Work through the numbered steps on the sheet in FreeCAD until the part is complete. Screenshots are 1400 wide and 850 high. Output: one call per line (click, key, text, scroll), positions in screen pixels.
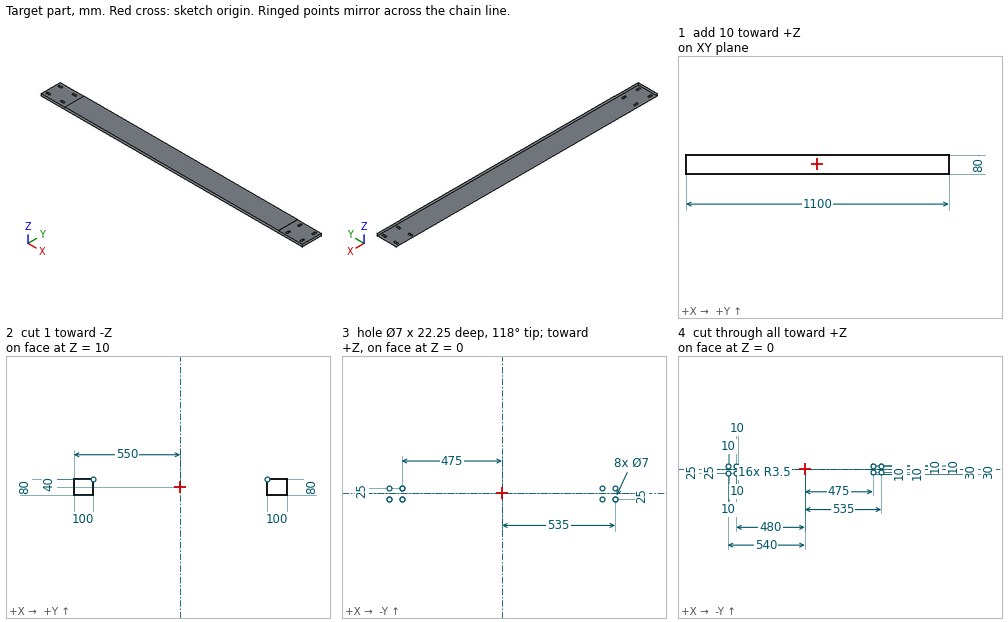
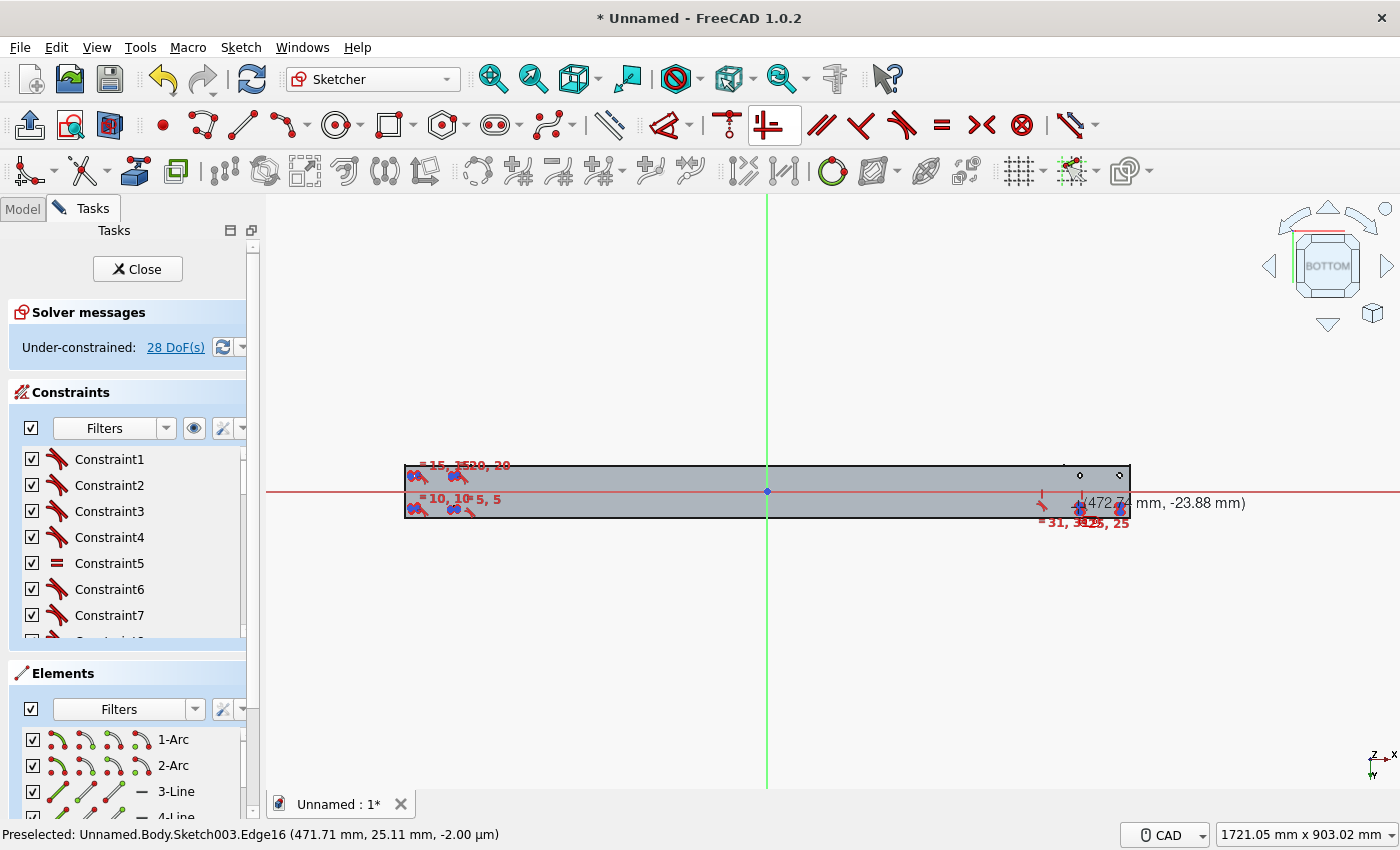
scroll(1120, 479, up, 12)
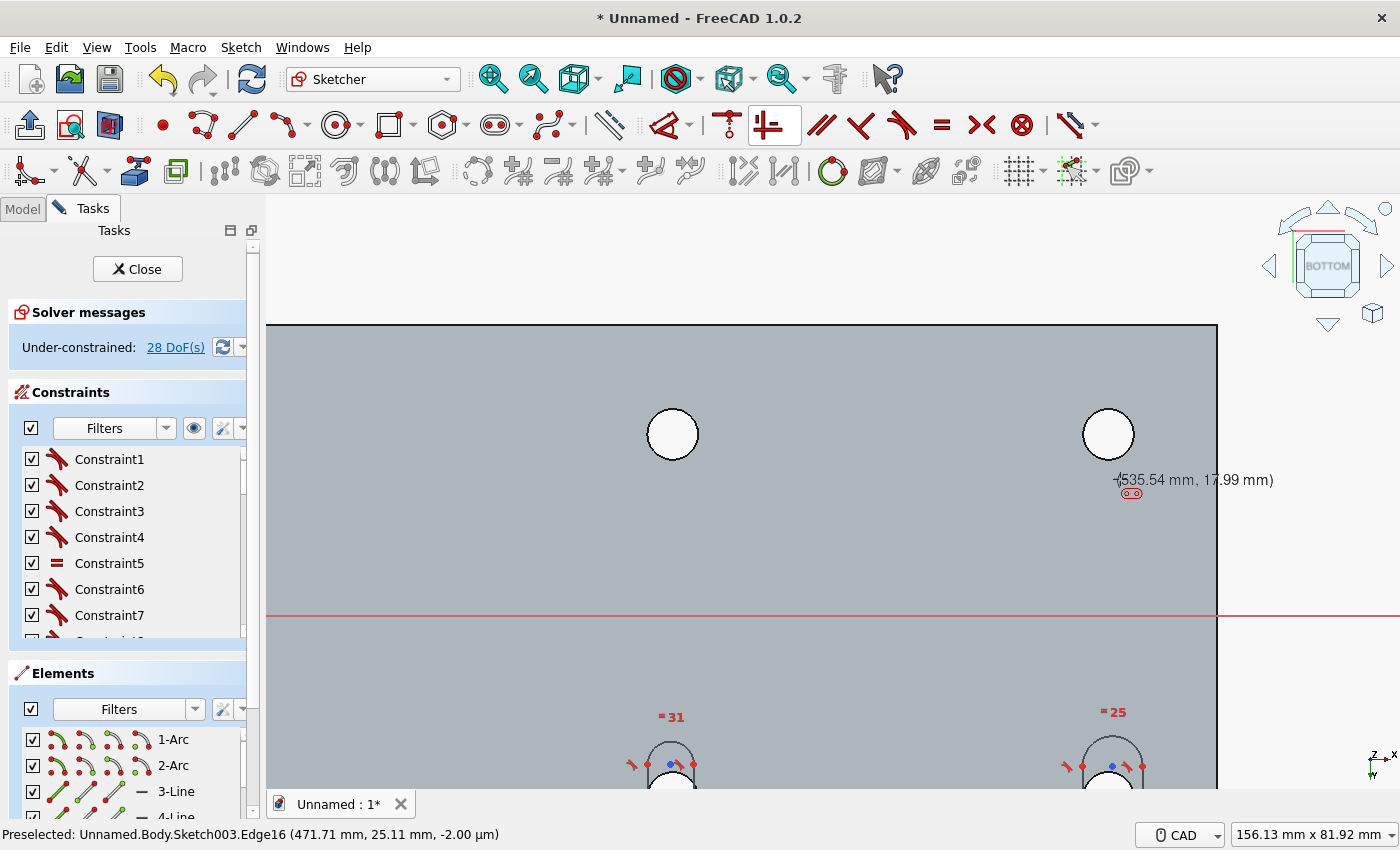
scroll(1120, 479, down, 12)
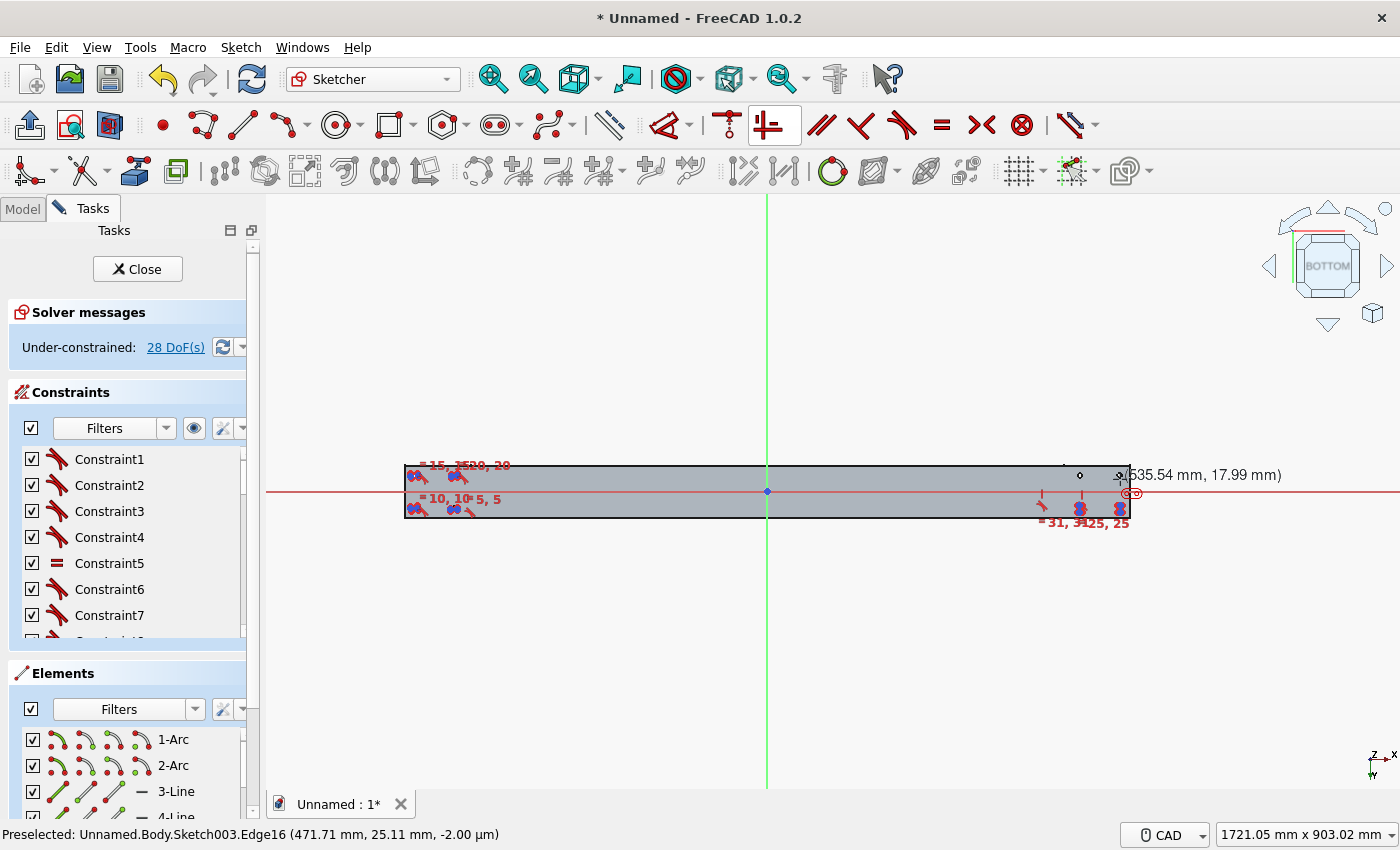
click(1120, 479)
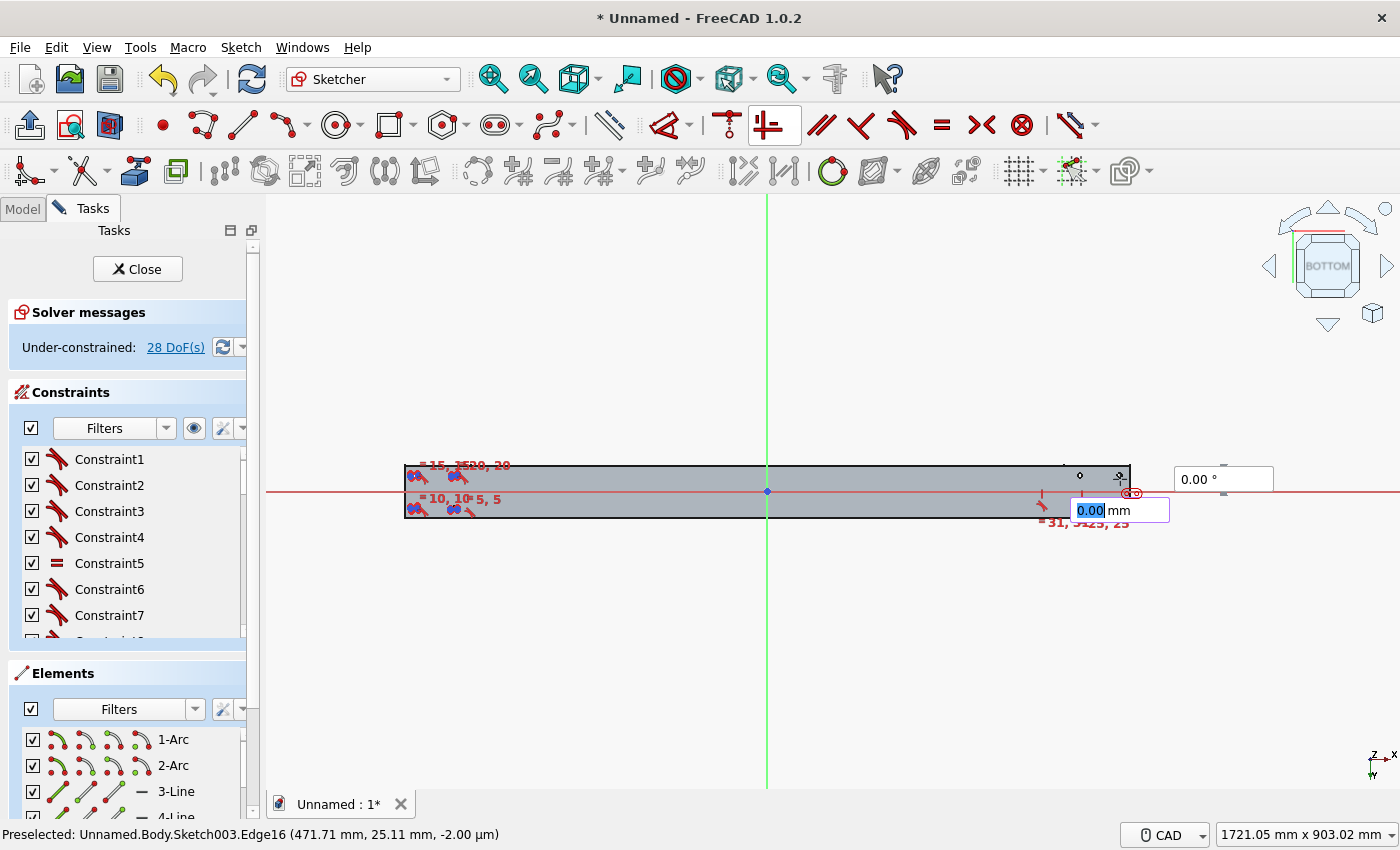
scroll(1120, 472, up, 5)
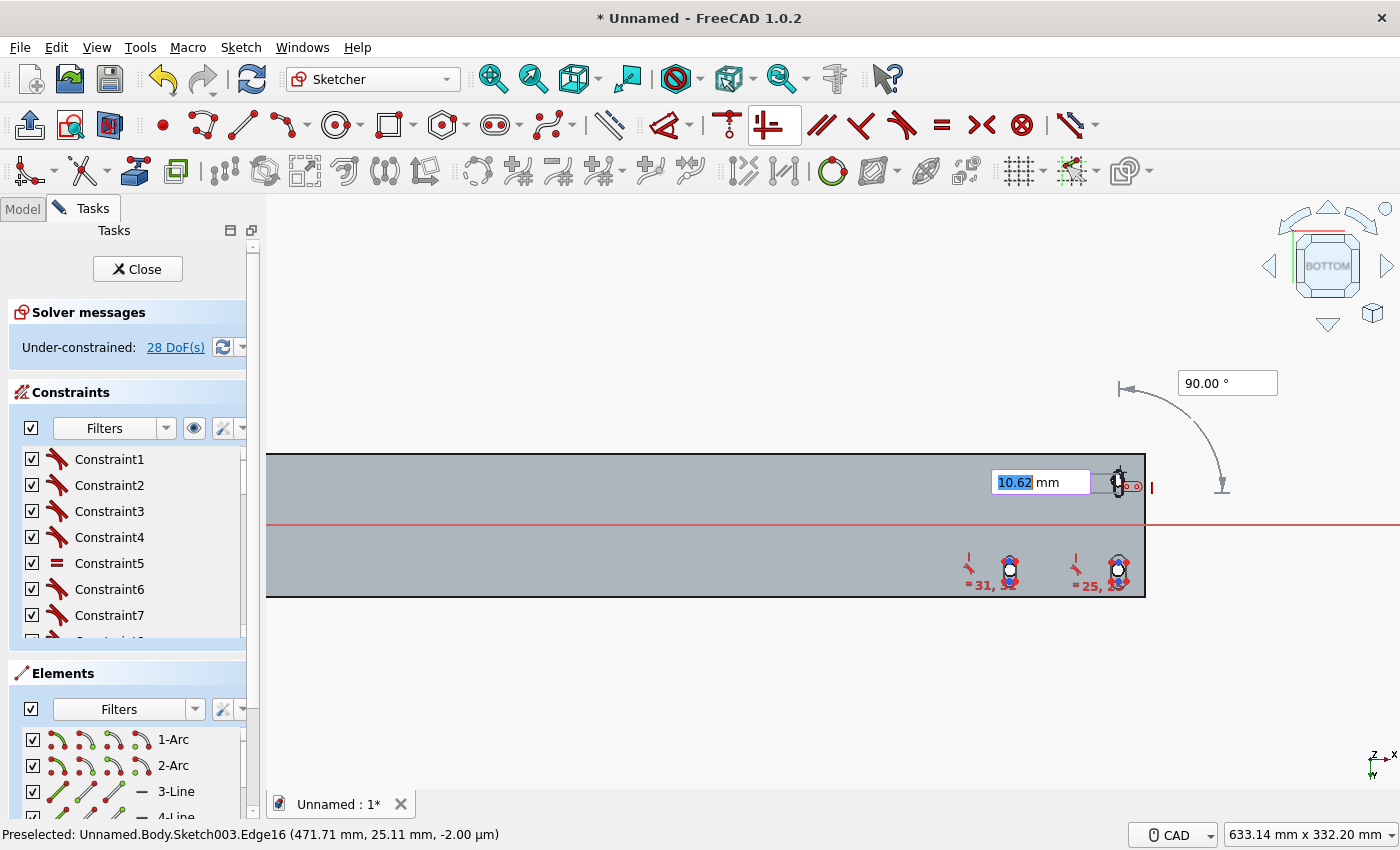
click(1119, 471)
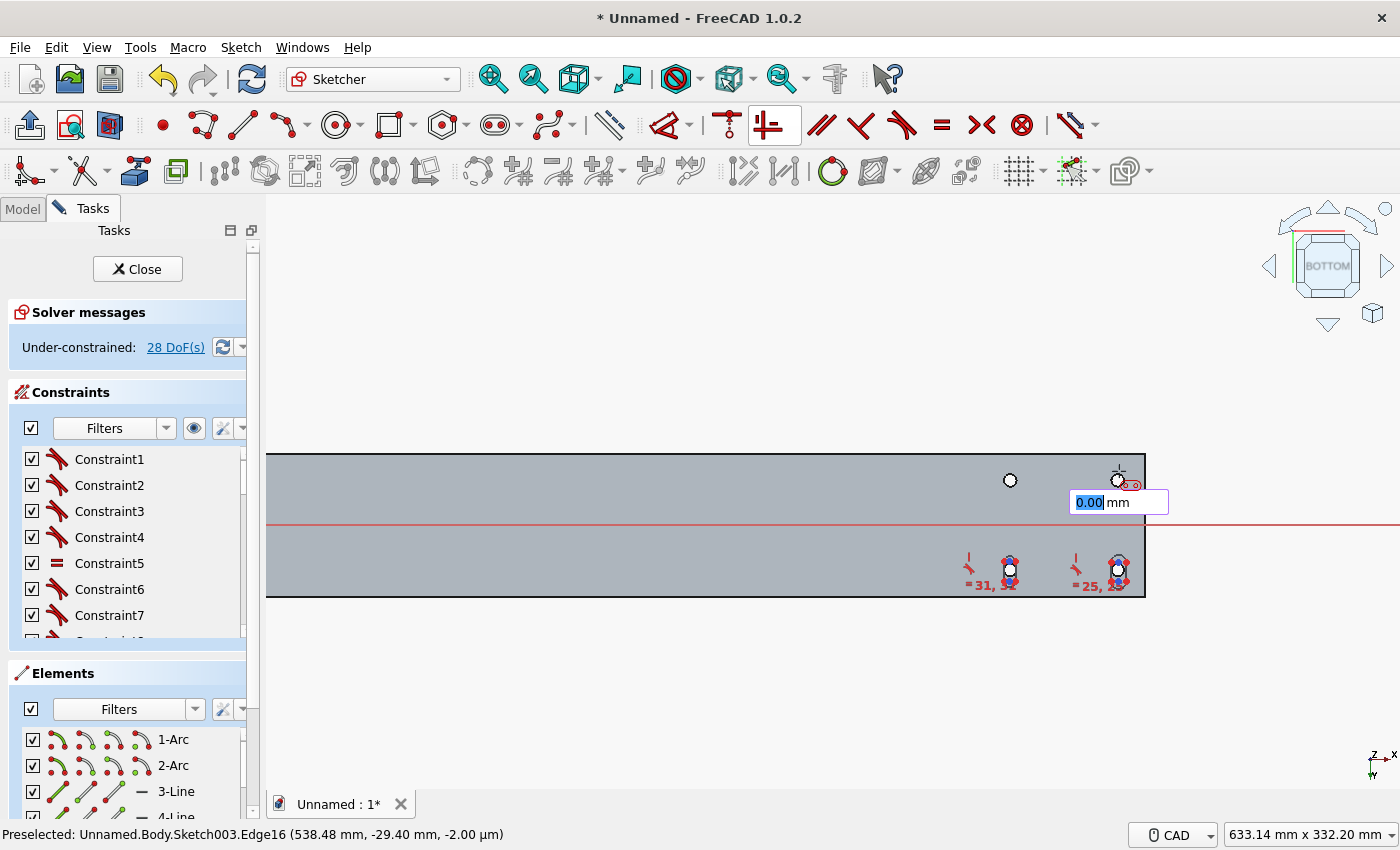
scroll(1124, 480, up, 5)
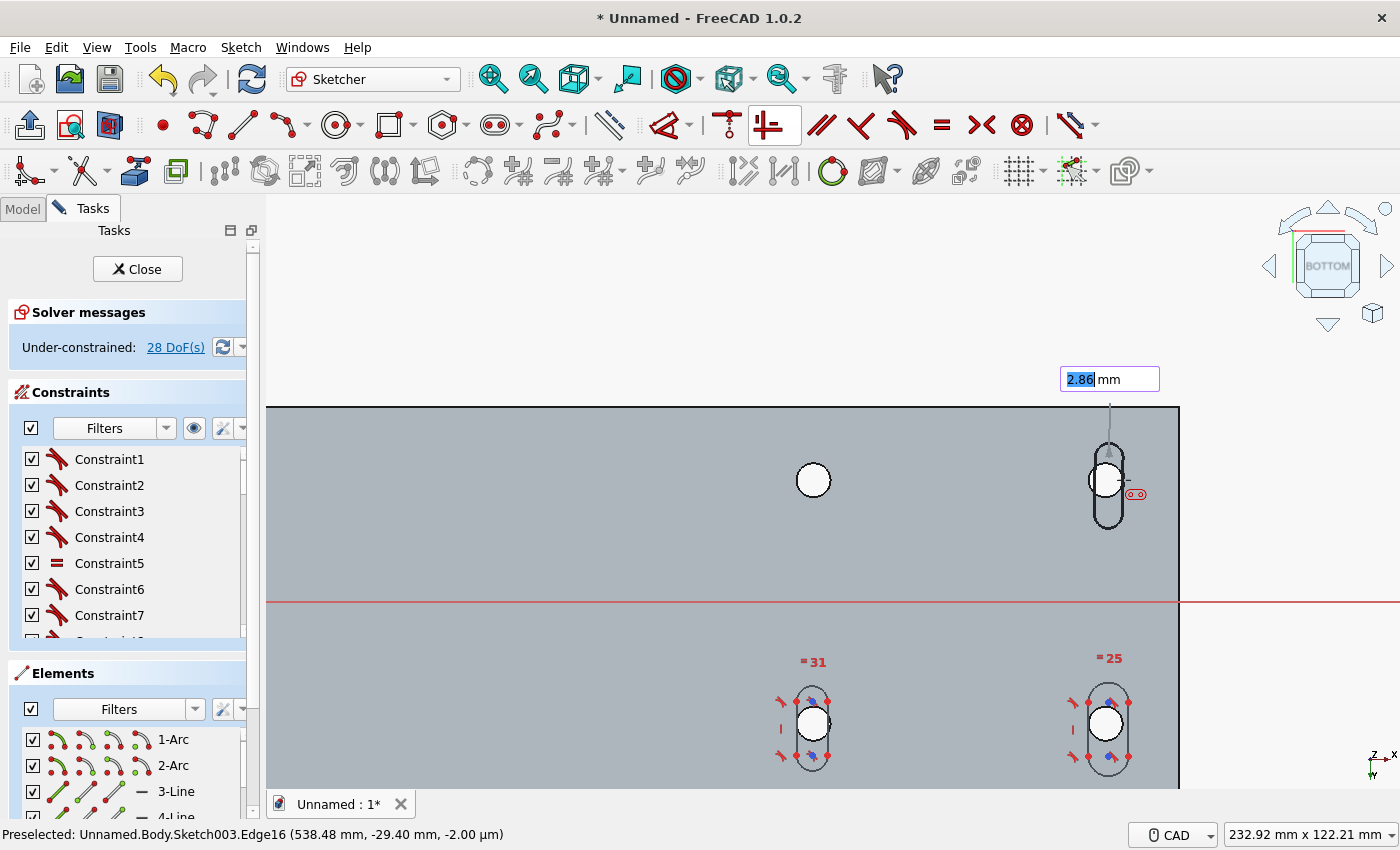
click(1123, 480)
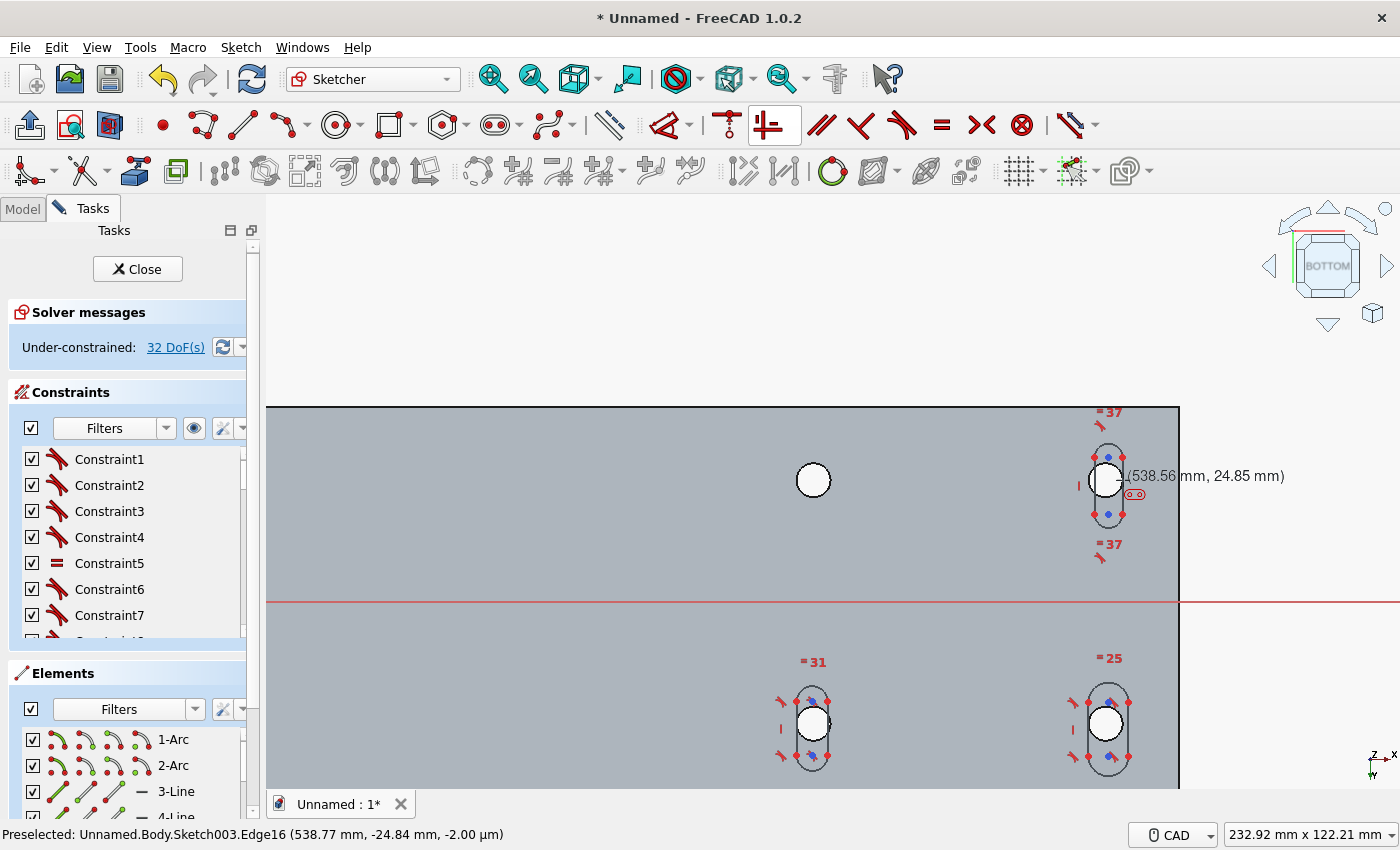
scroll(814, 505, up, 2)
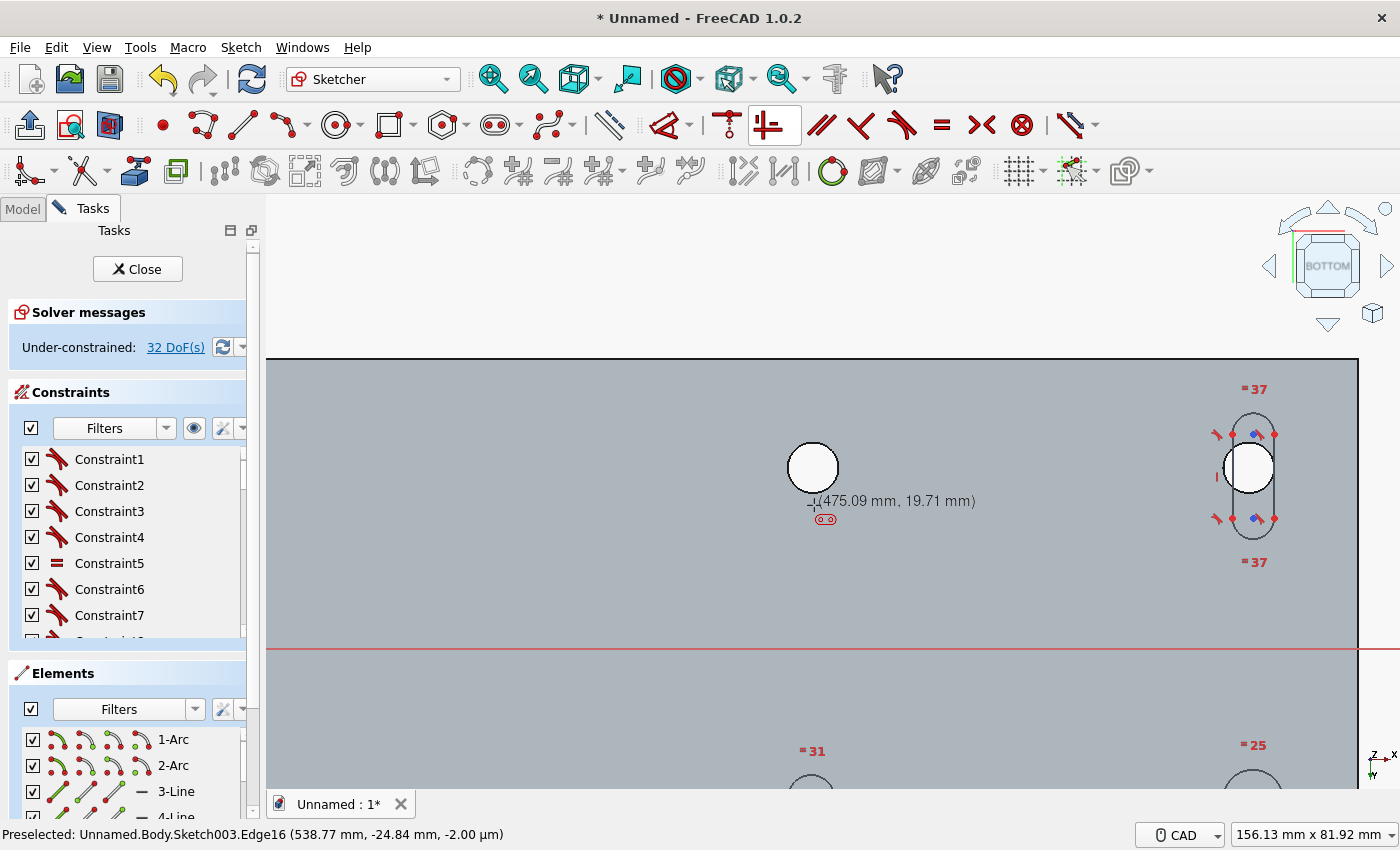
scroll(1106, 476, down, 12)